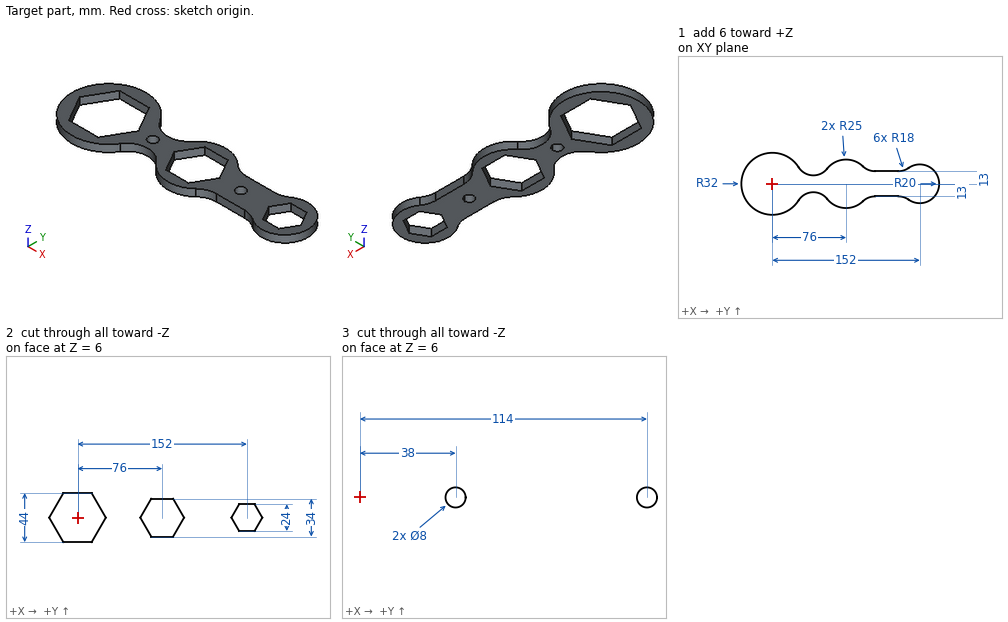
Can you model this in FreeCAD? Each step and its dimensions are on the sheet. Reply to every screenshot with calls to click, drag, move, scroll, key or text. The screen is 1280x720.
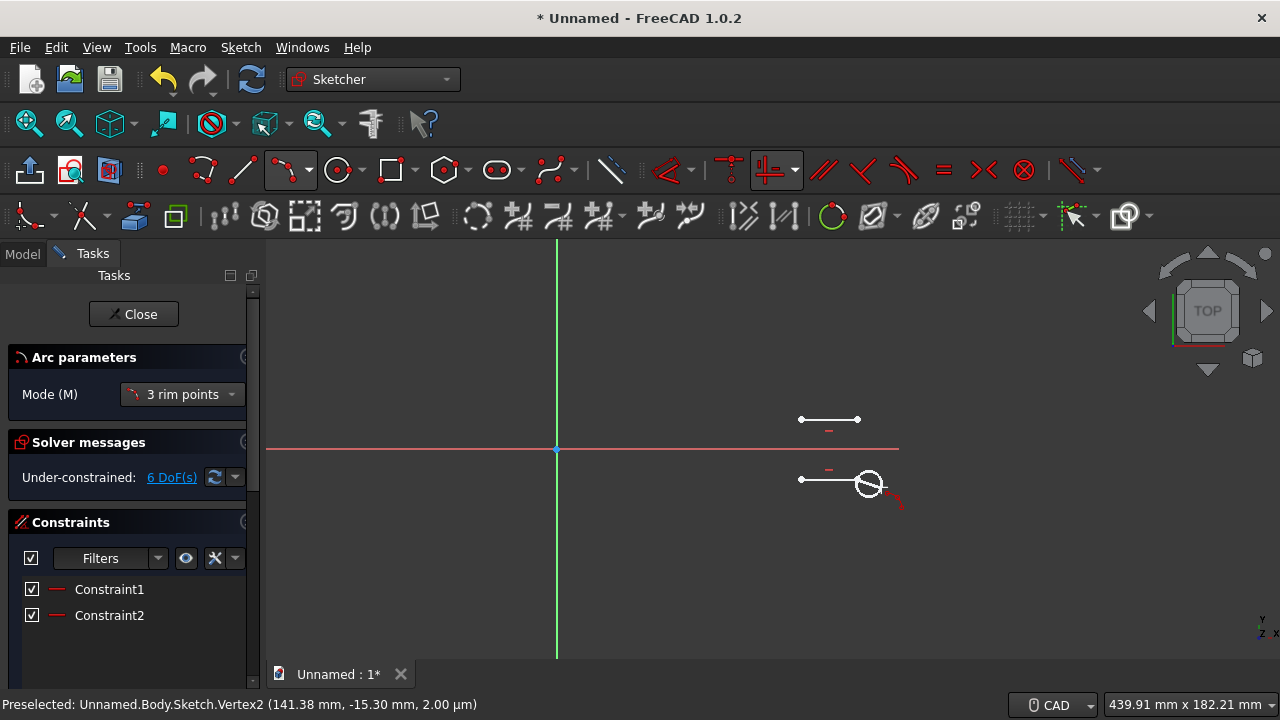
scroll(869, 481, up, 11)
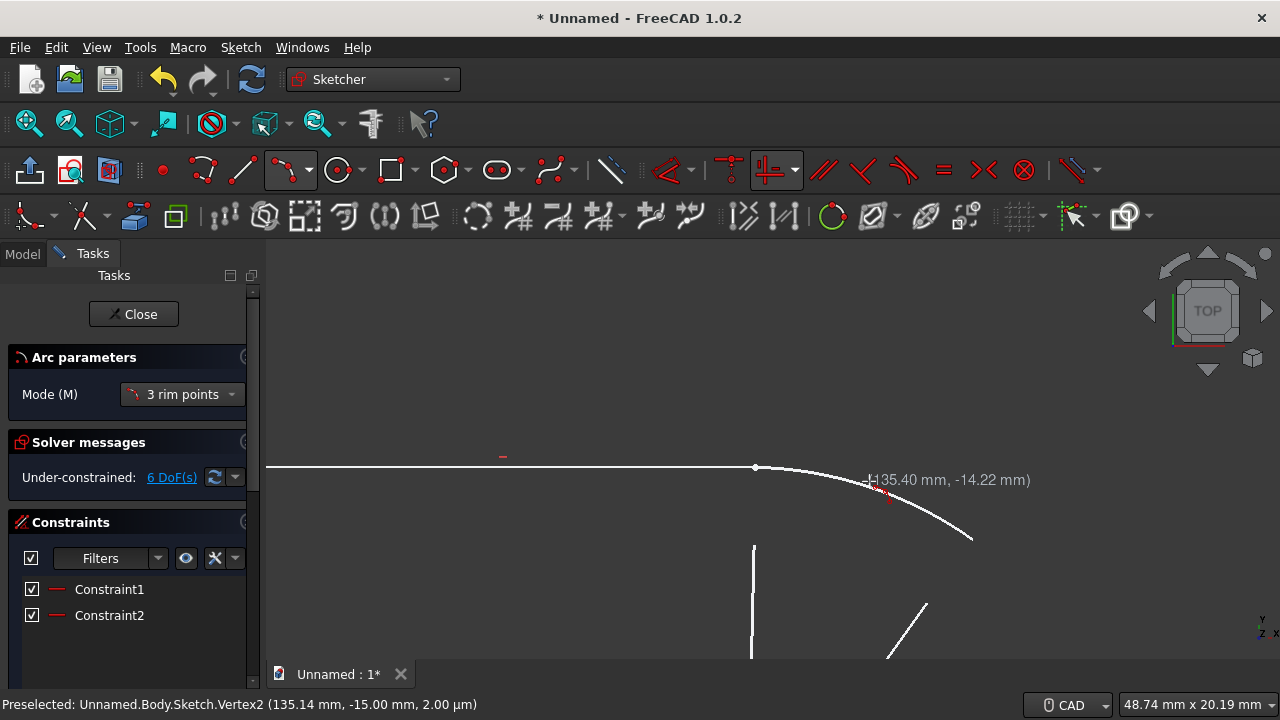
click(866, 478)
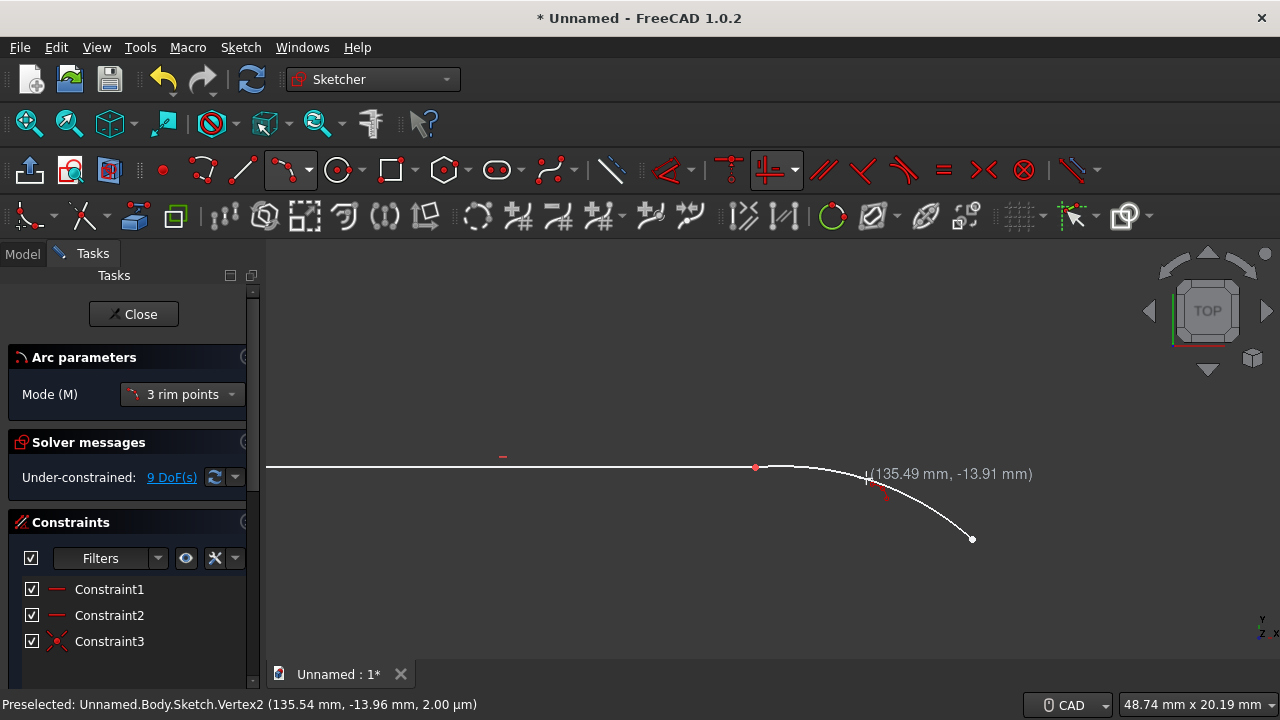
scroll(892, 490, down, 10)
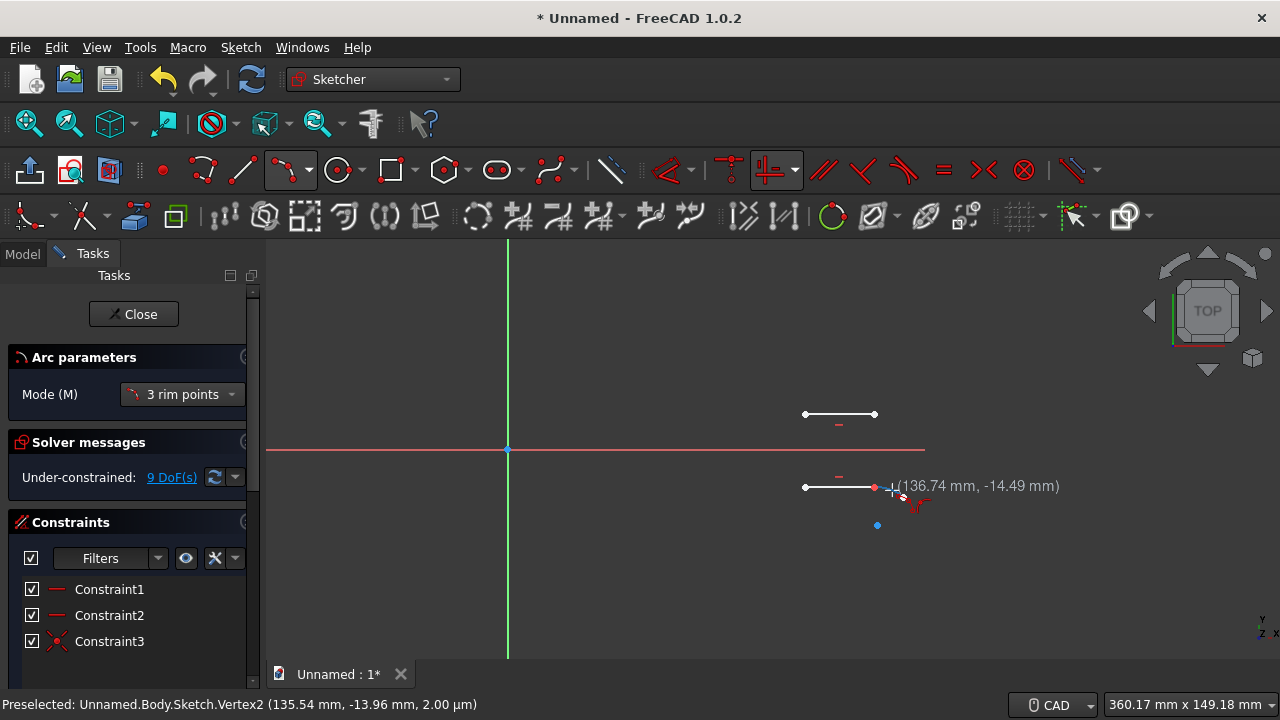
click(903, 497)
click(903, 404)
click(987, 474)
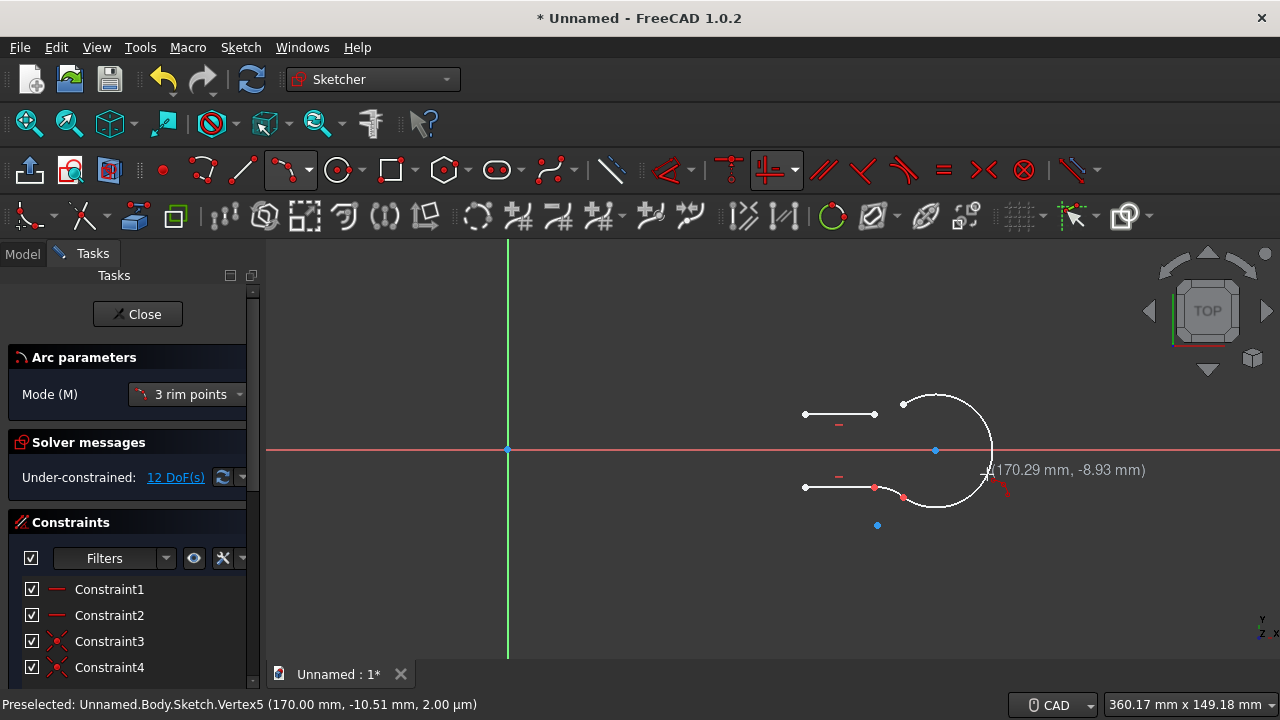
click(903, 405)
click(874, 414)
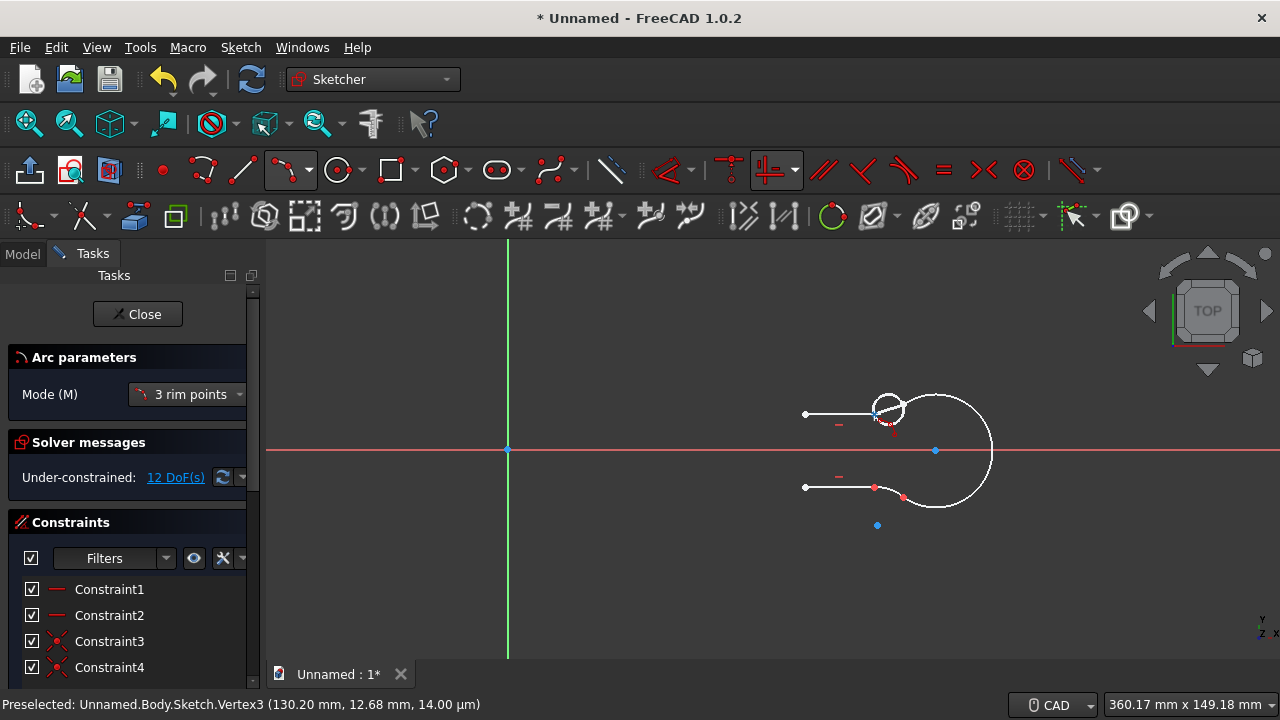
scroll(889, 411, up, 10)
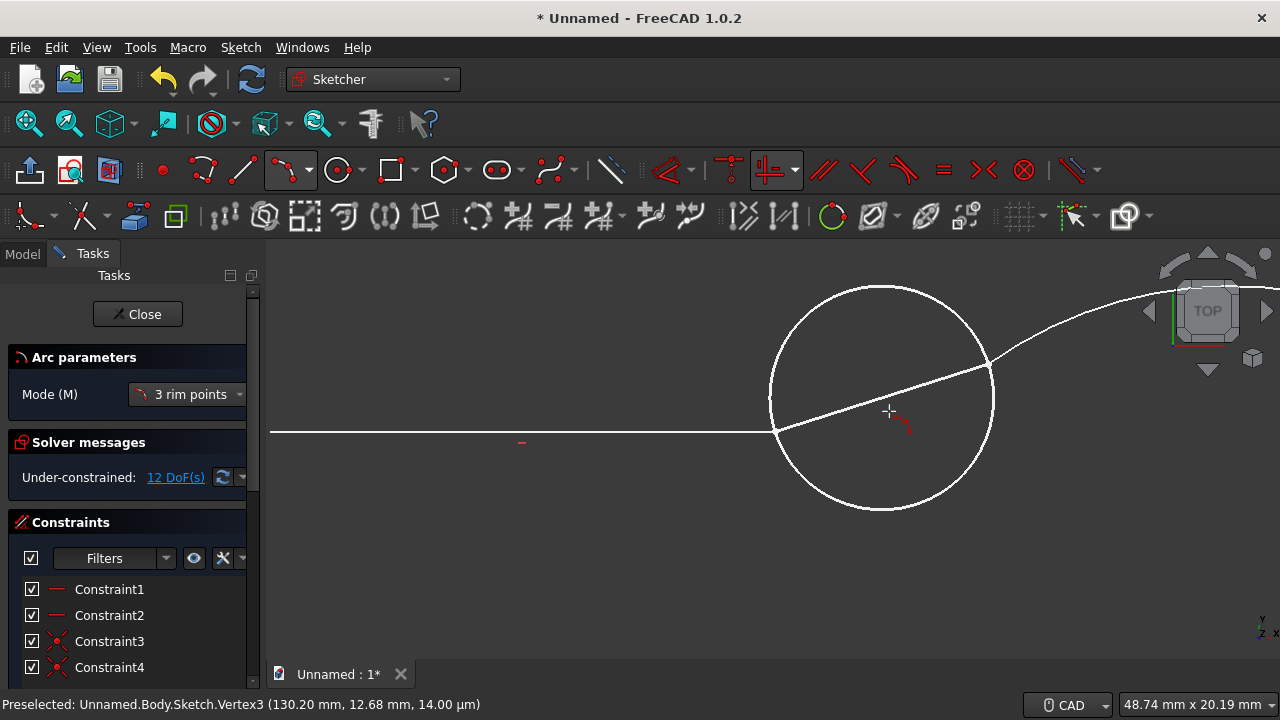
click(885, 407)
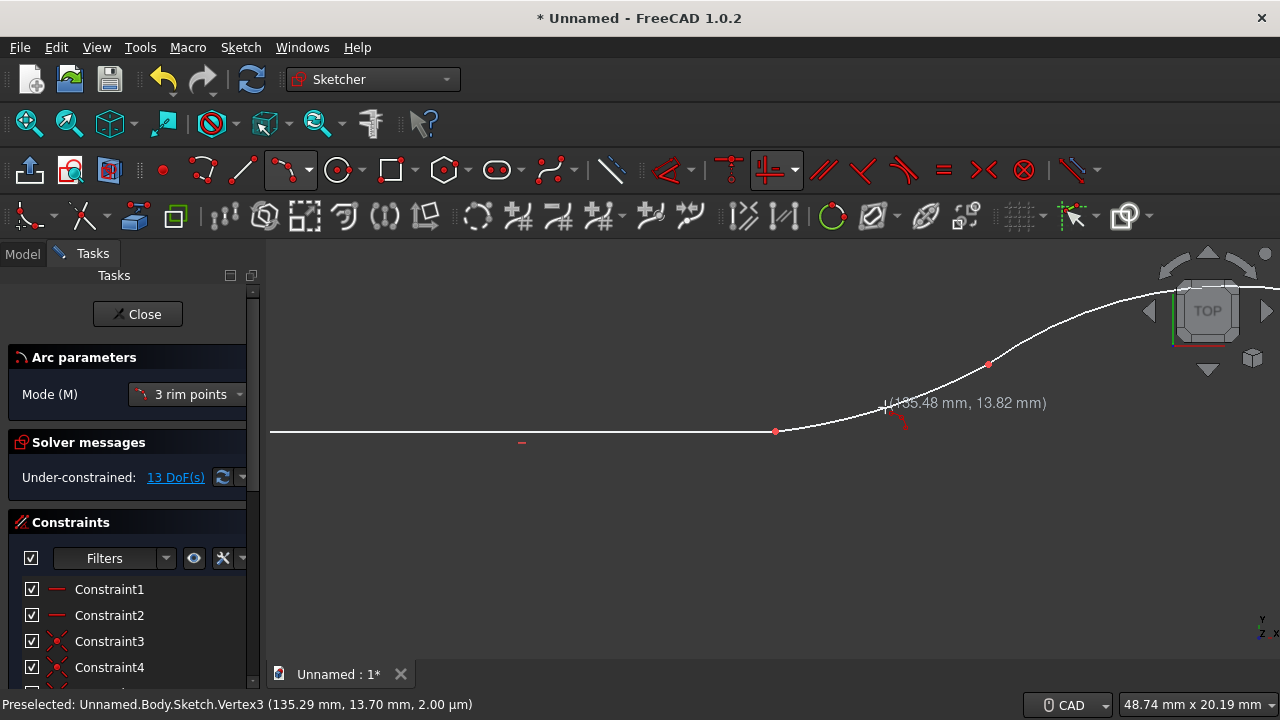
scroll(889, 410, down, 10)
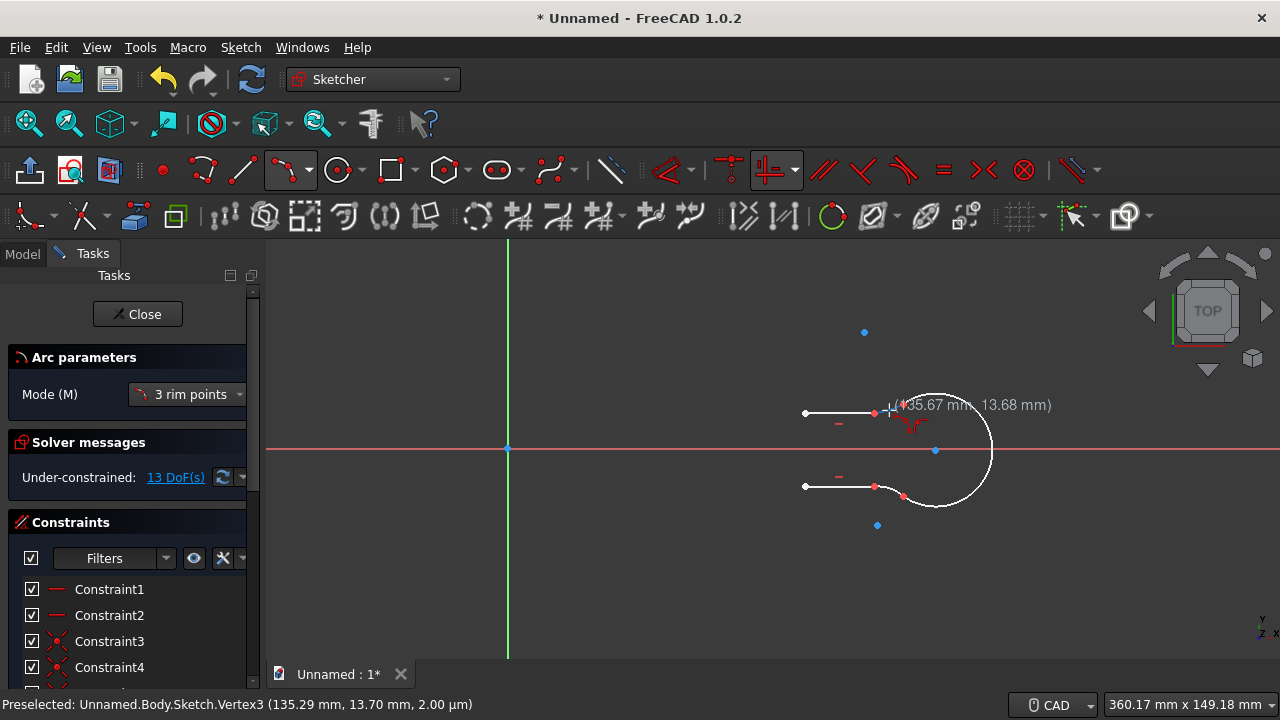
click(806, 413)
click(770, 398)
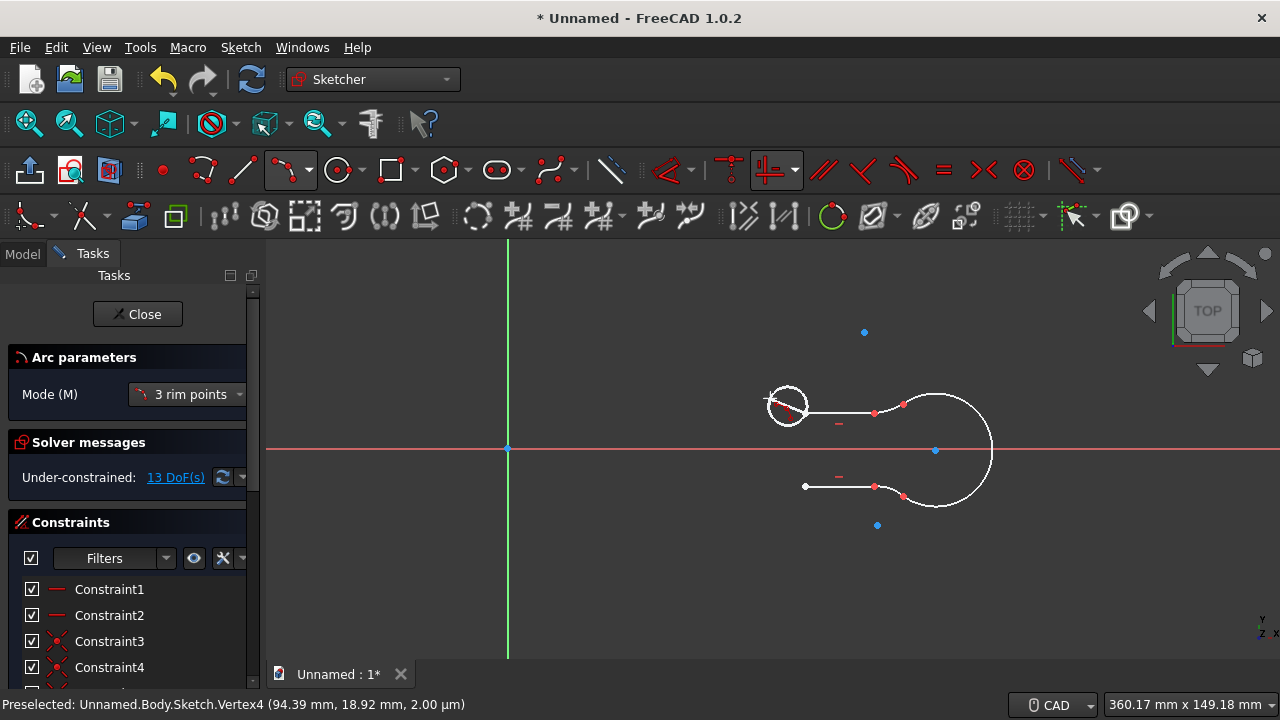
scroll(786, 409, up, 8)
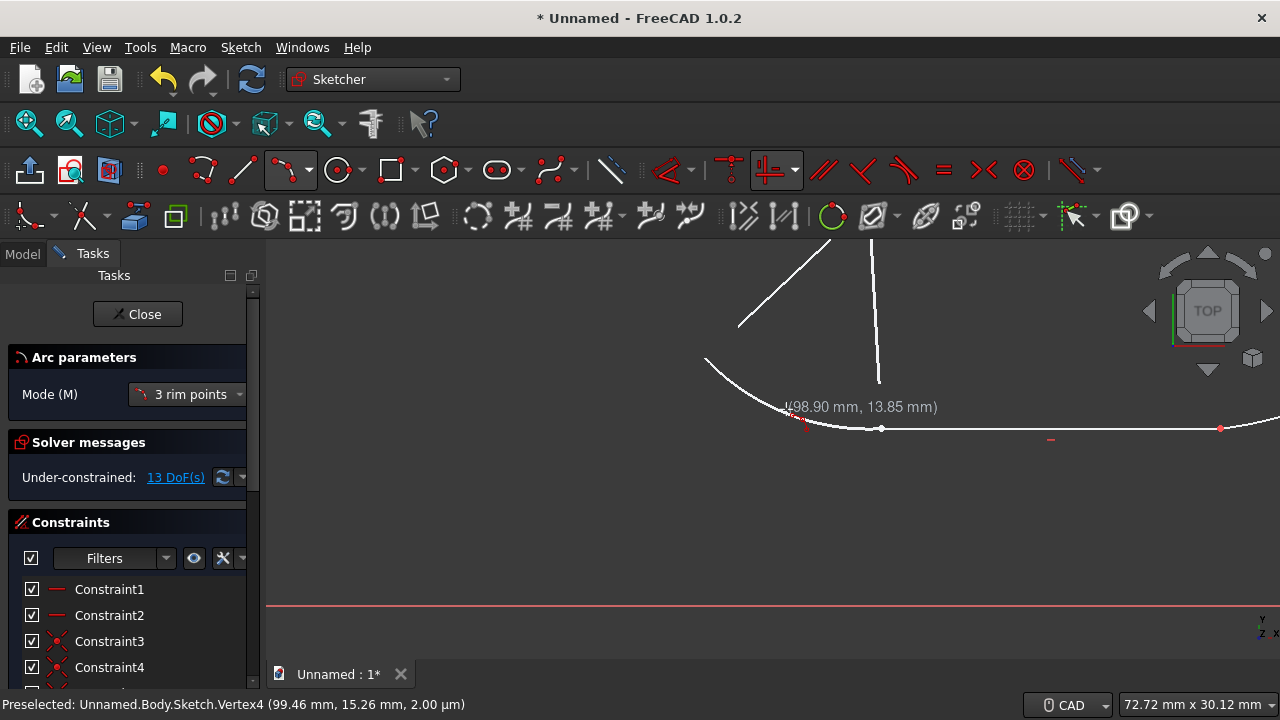
click(786, 406)